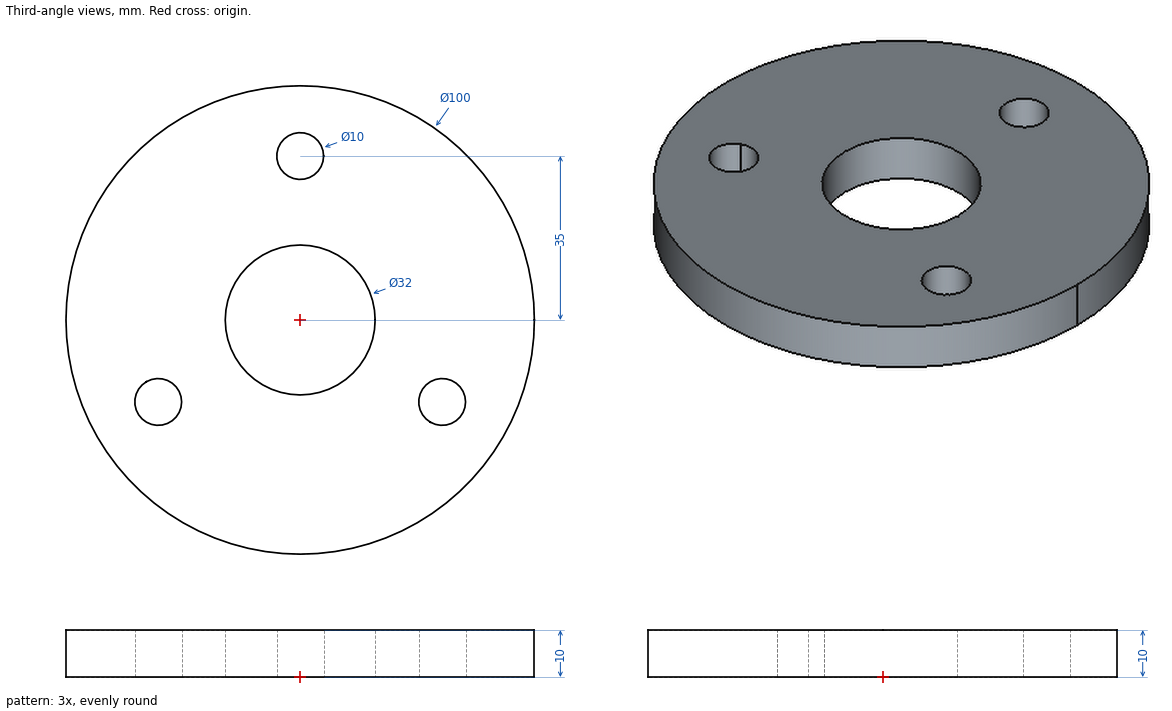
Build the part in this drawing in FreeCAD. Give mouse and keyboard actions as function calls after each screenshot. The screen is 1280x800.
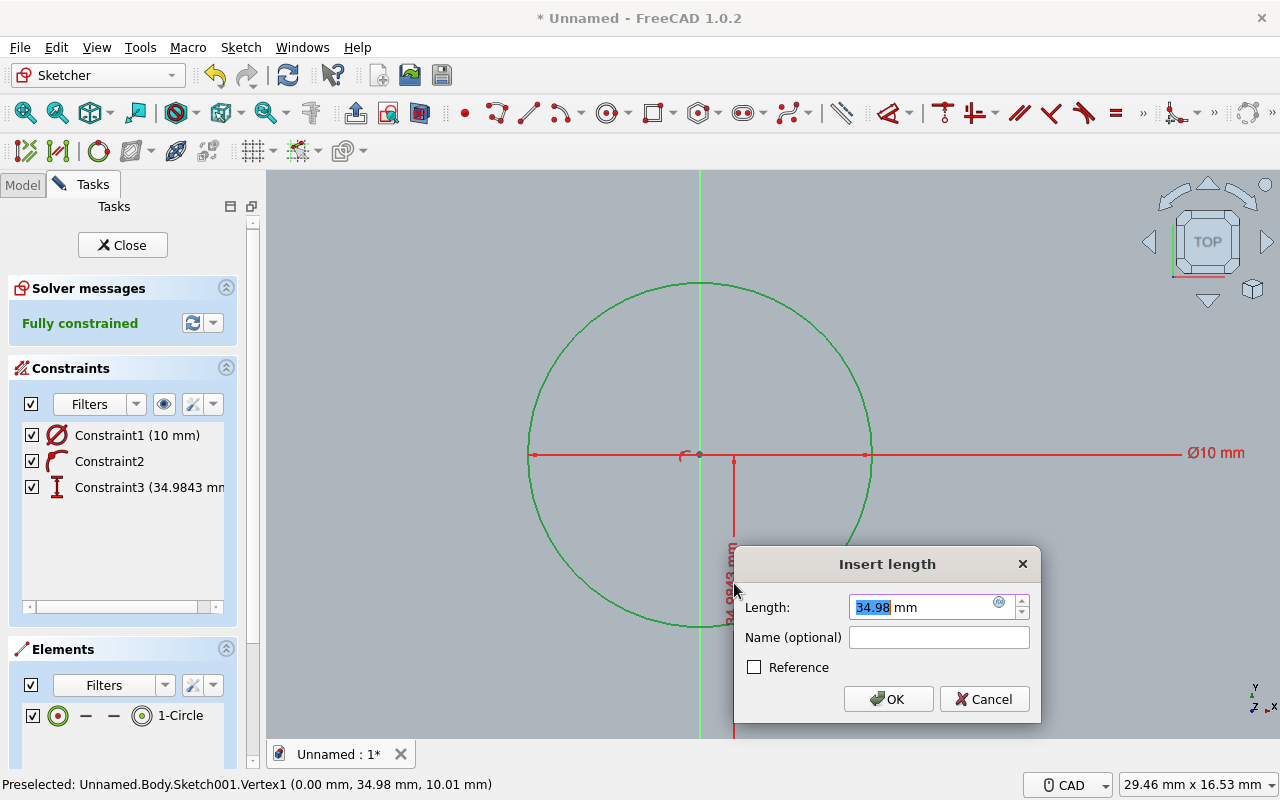
text(35)
key(Return)
key(Escape)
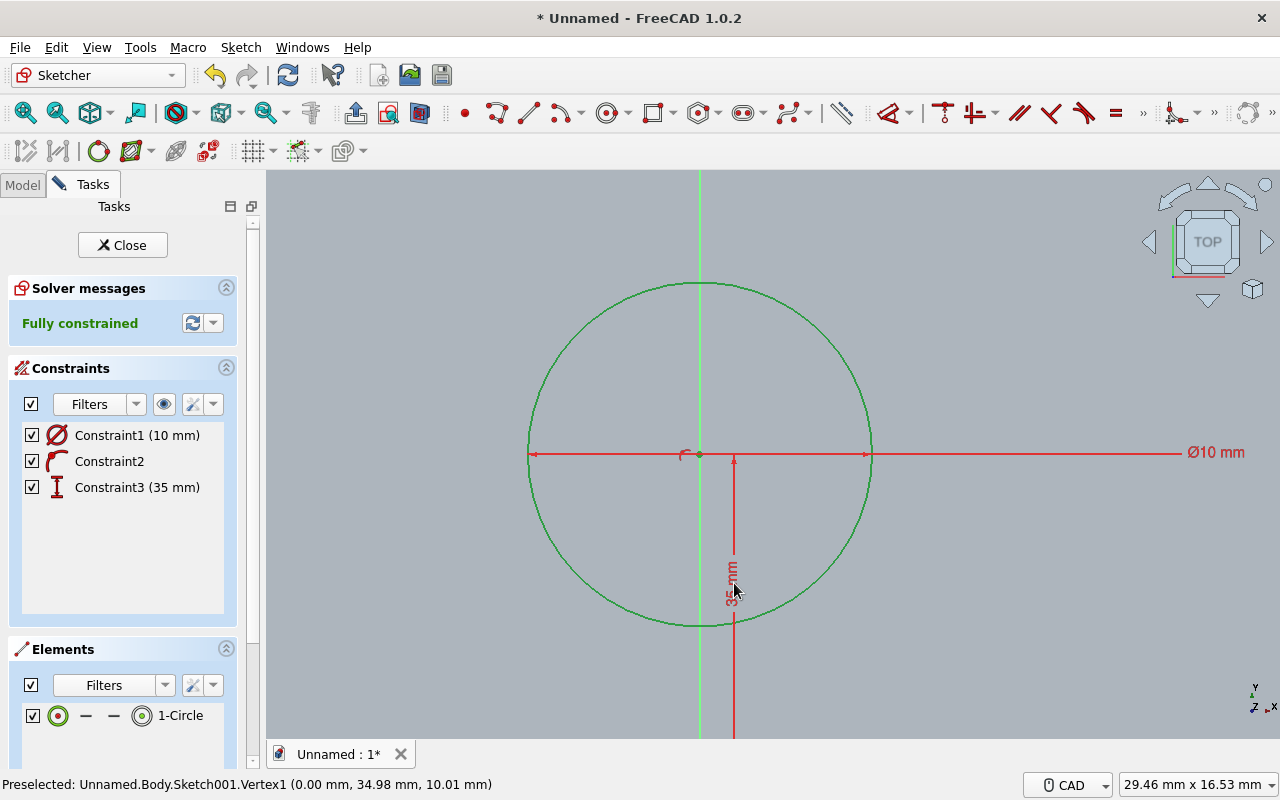
click(123, 245)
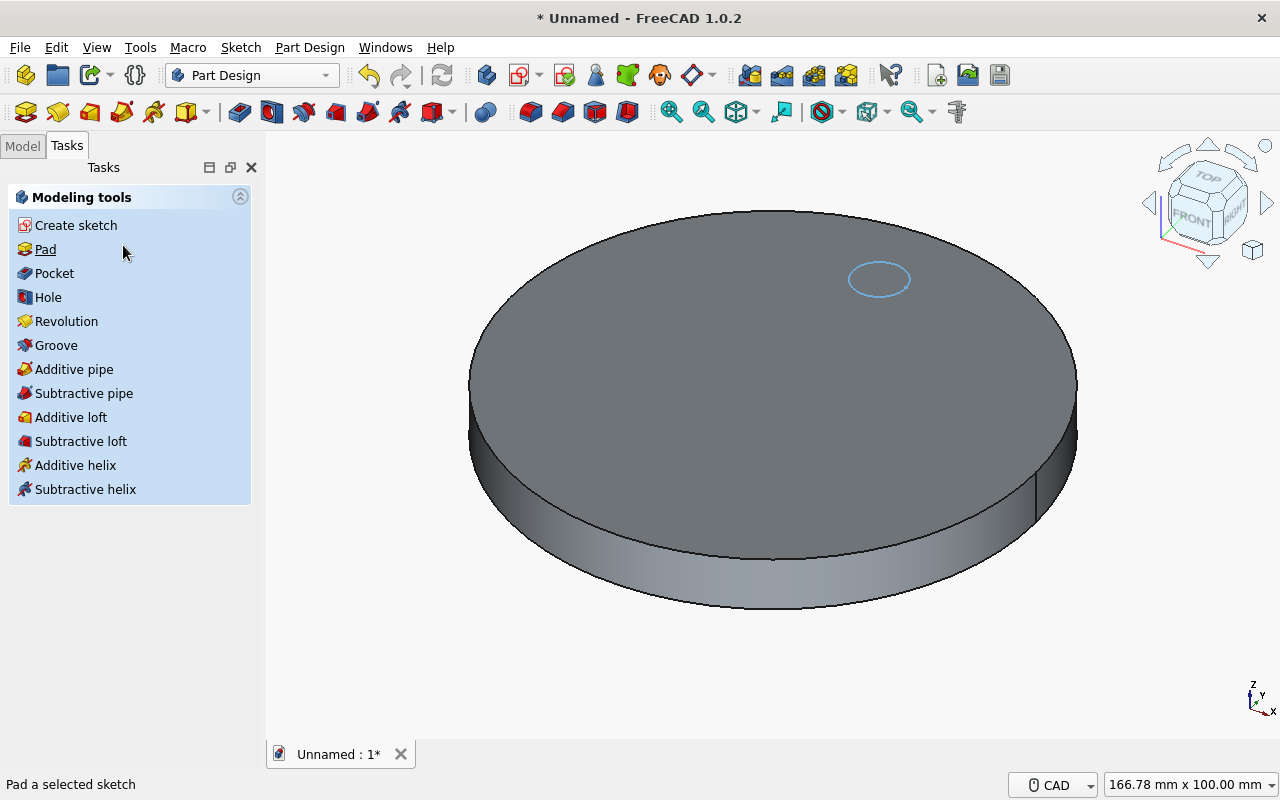
click(240, 112)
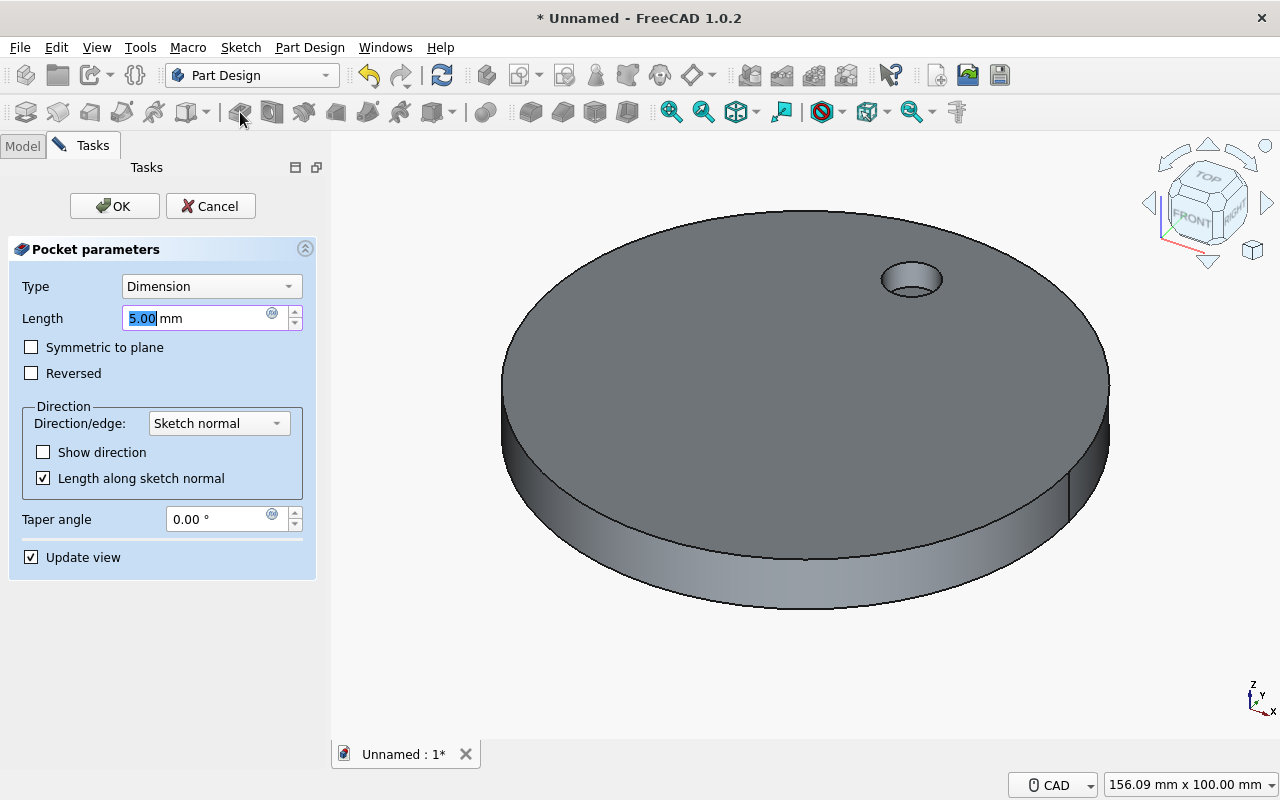
text(10)
key(Tab)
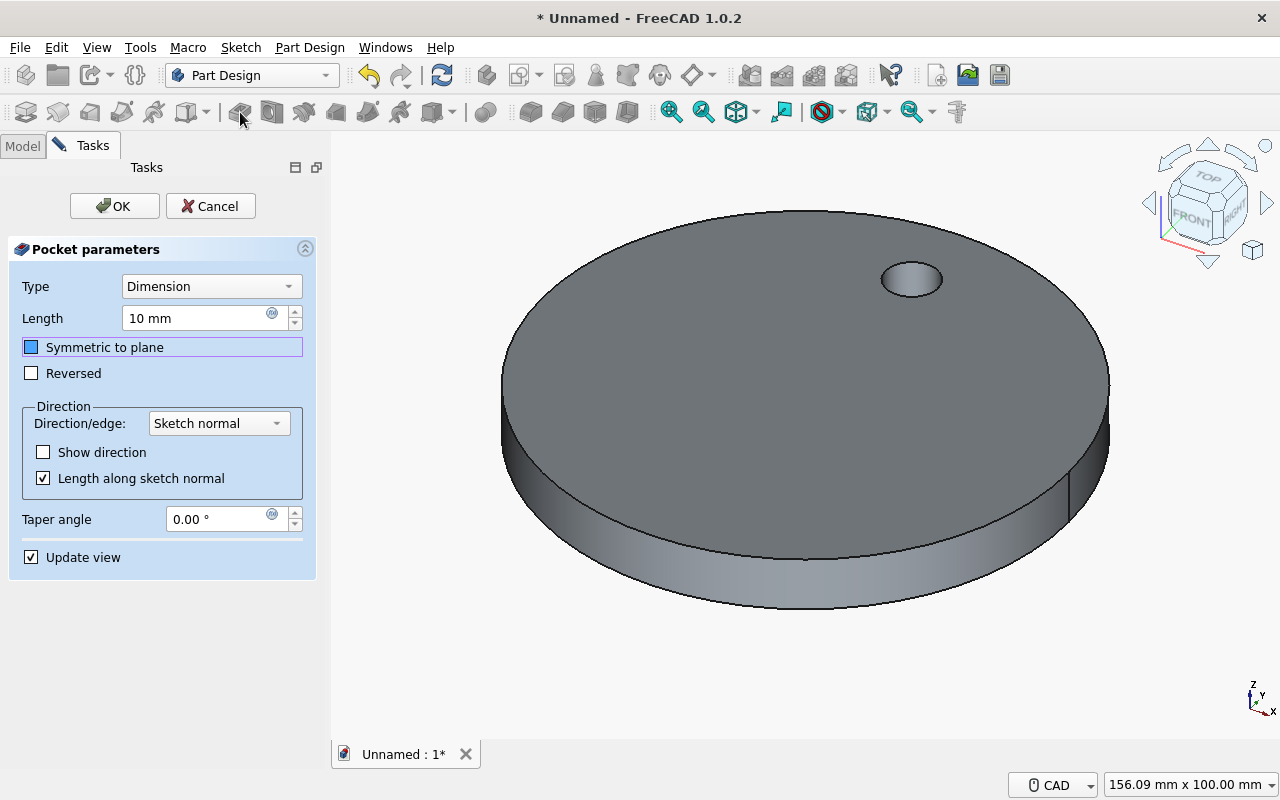
click(115, 206)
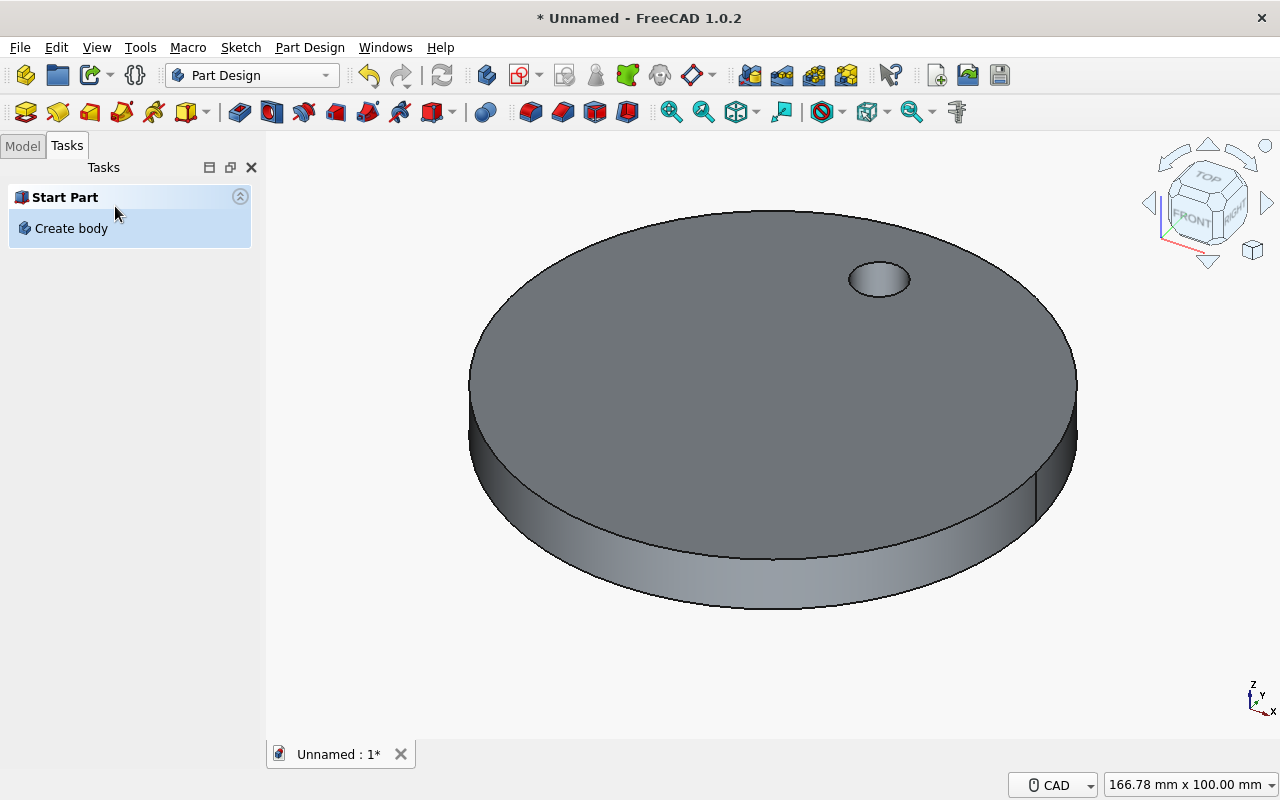
click(23, 145)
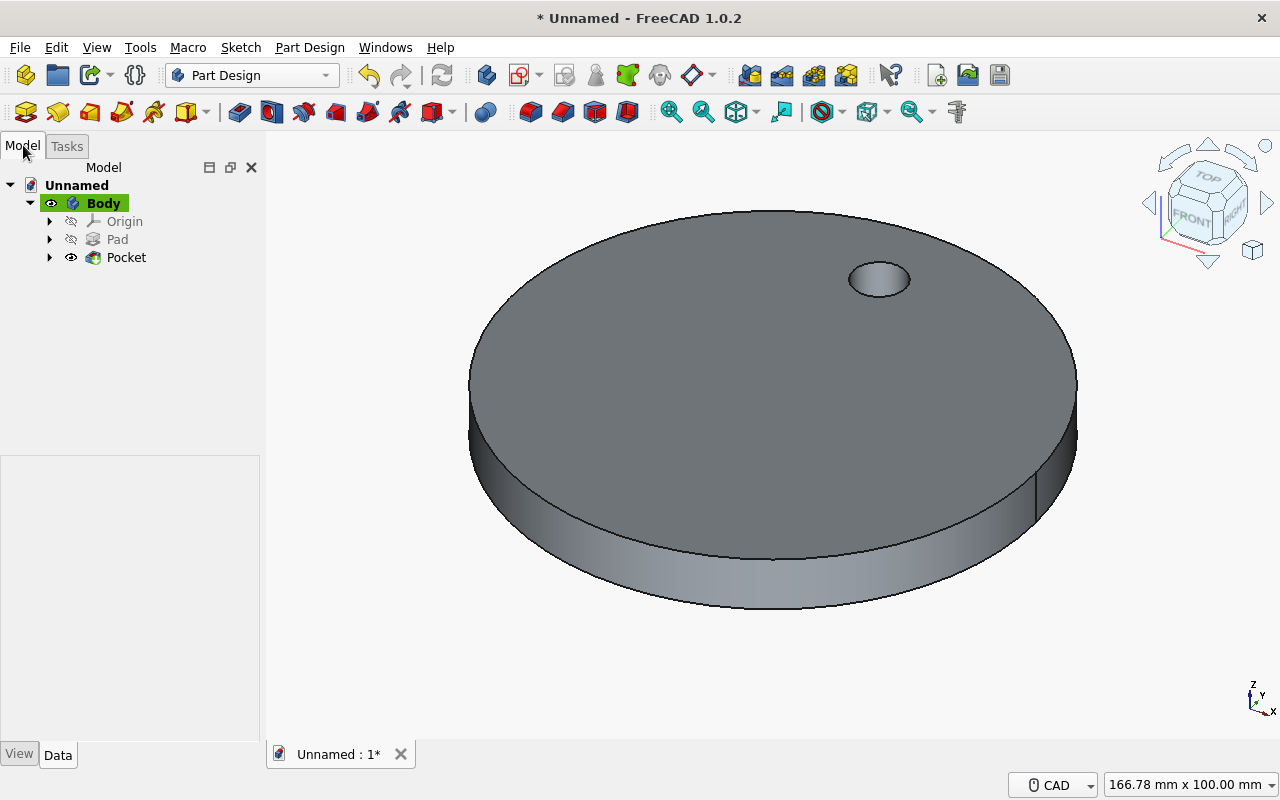
click(116, 257)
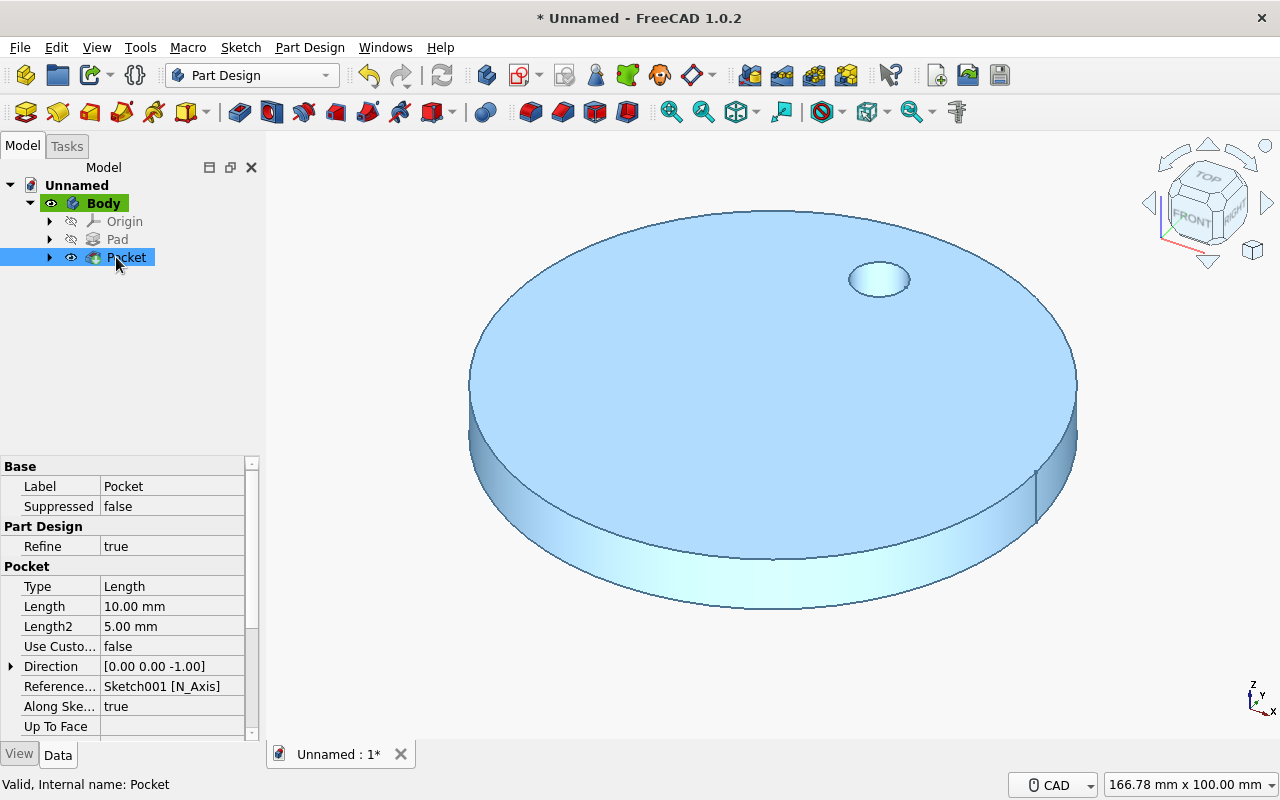
click(814, 76)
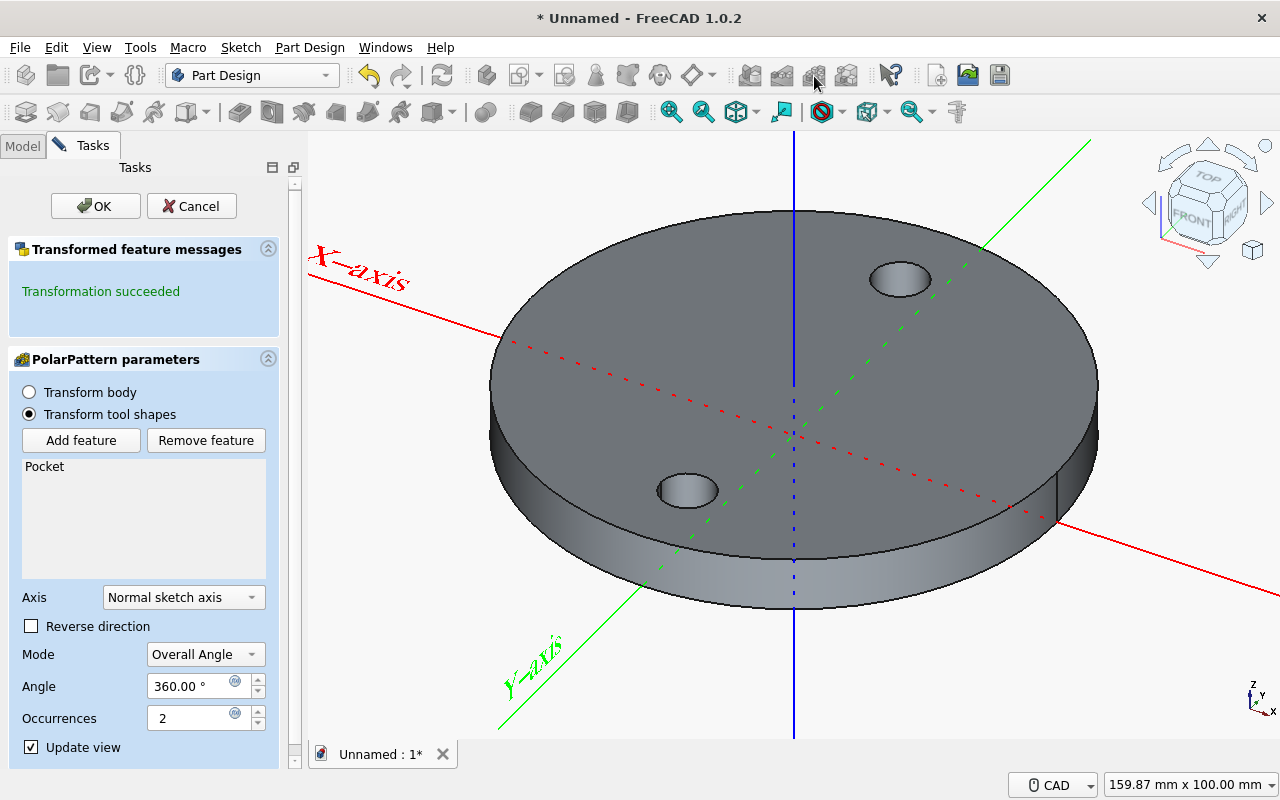
click(184, 598)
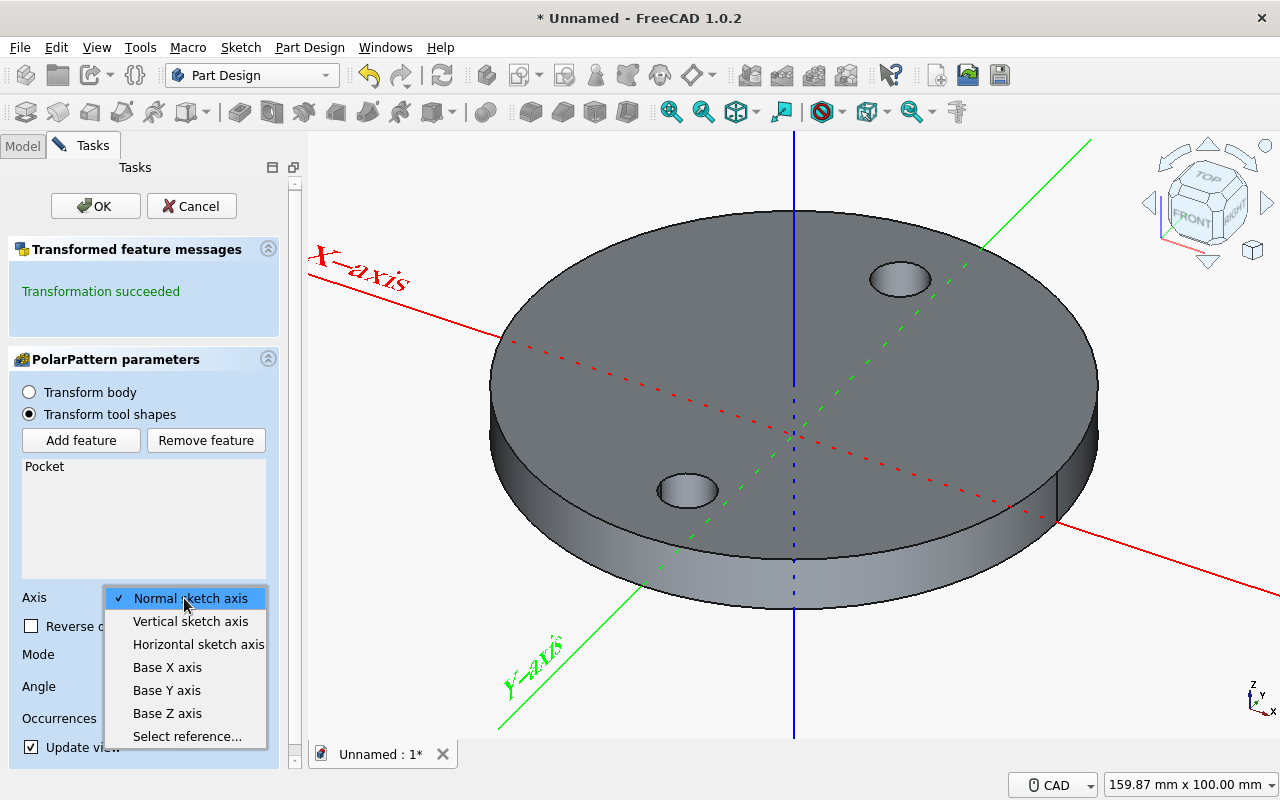
click(184, 714)